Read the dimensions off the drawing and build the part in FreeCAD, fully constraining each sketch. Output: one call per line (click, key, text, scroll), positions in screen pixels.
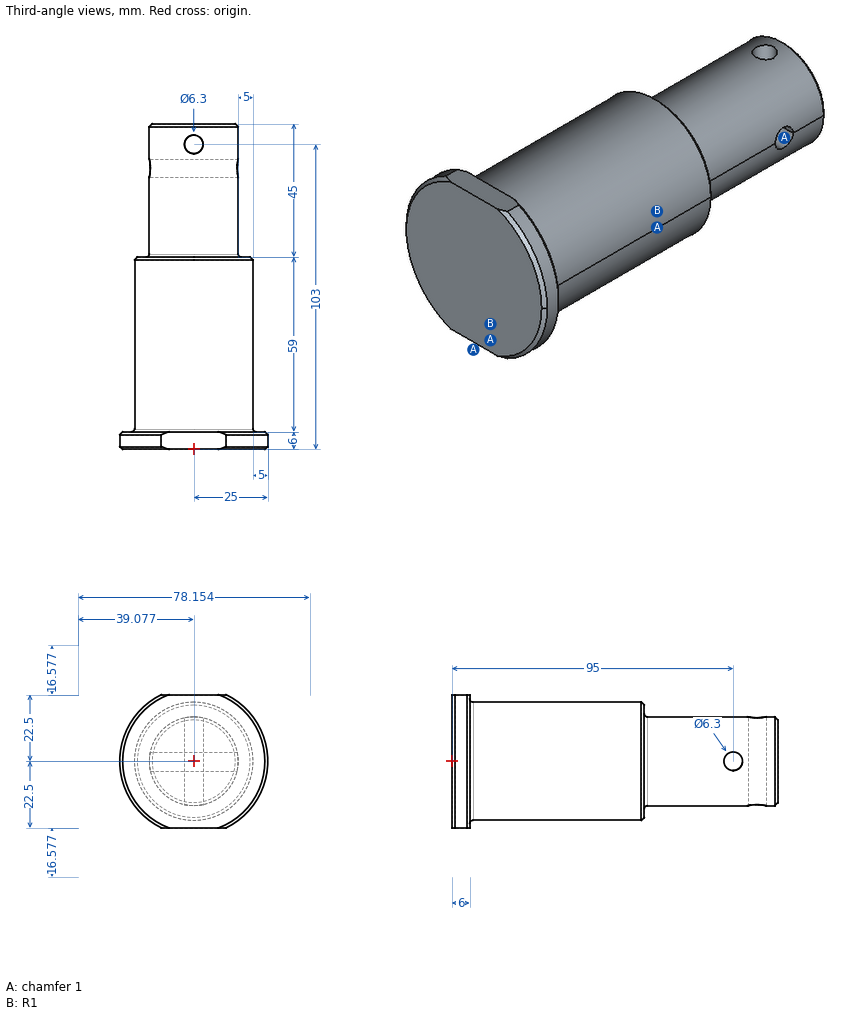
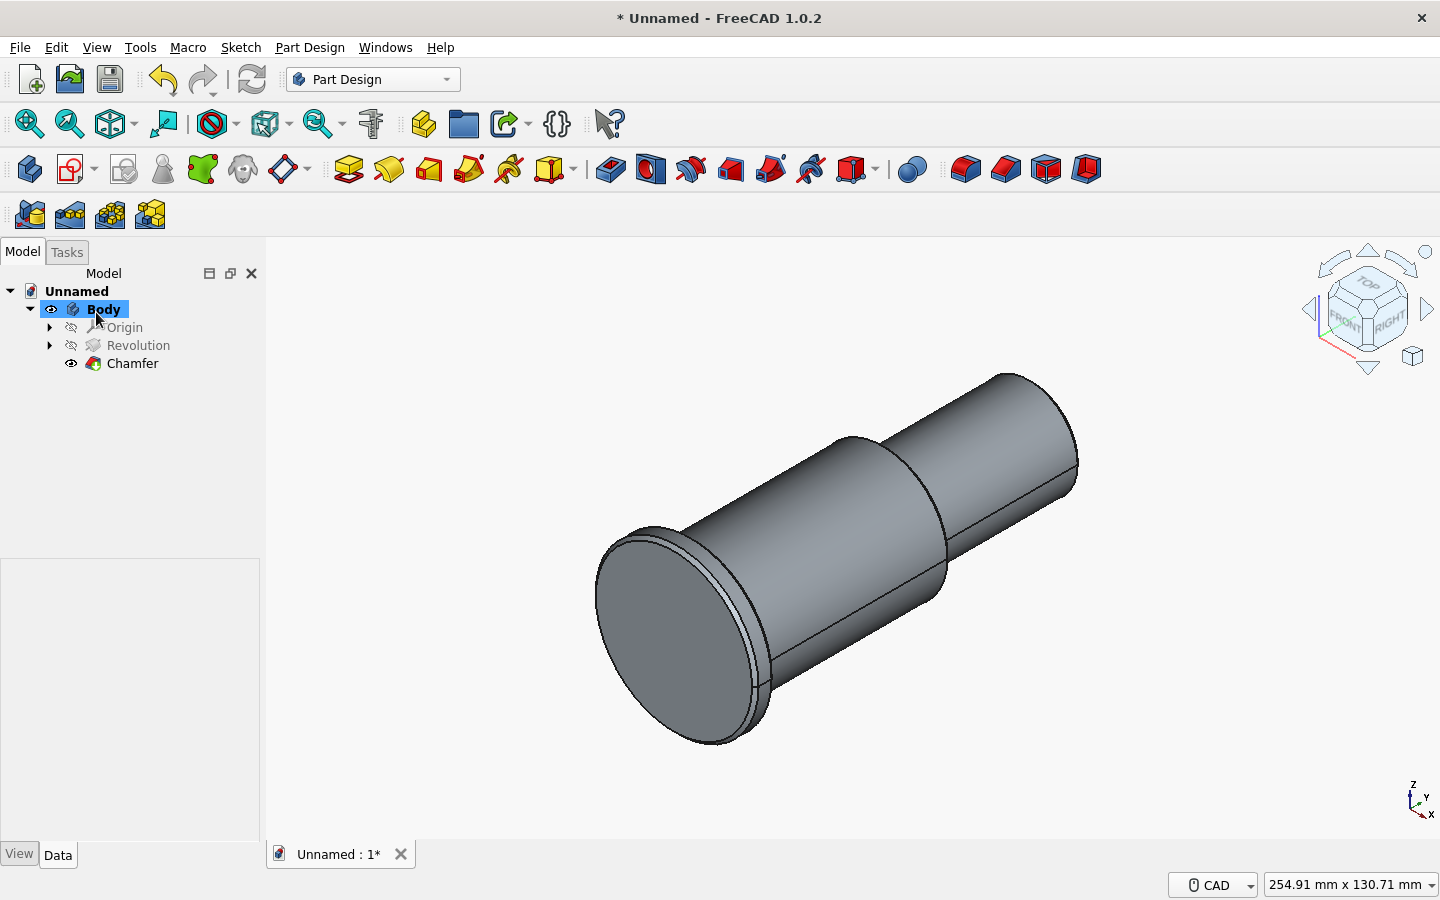
key(2)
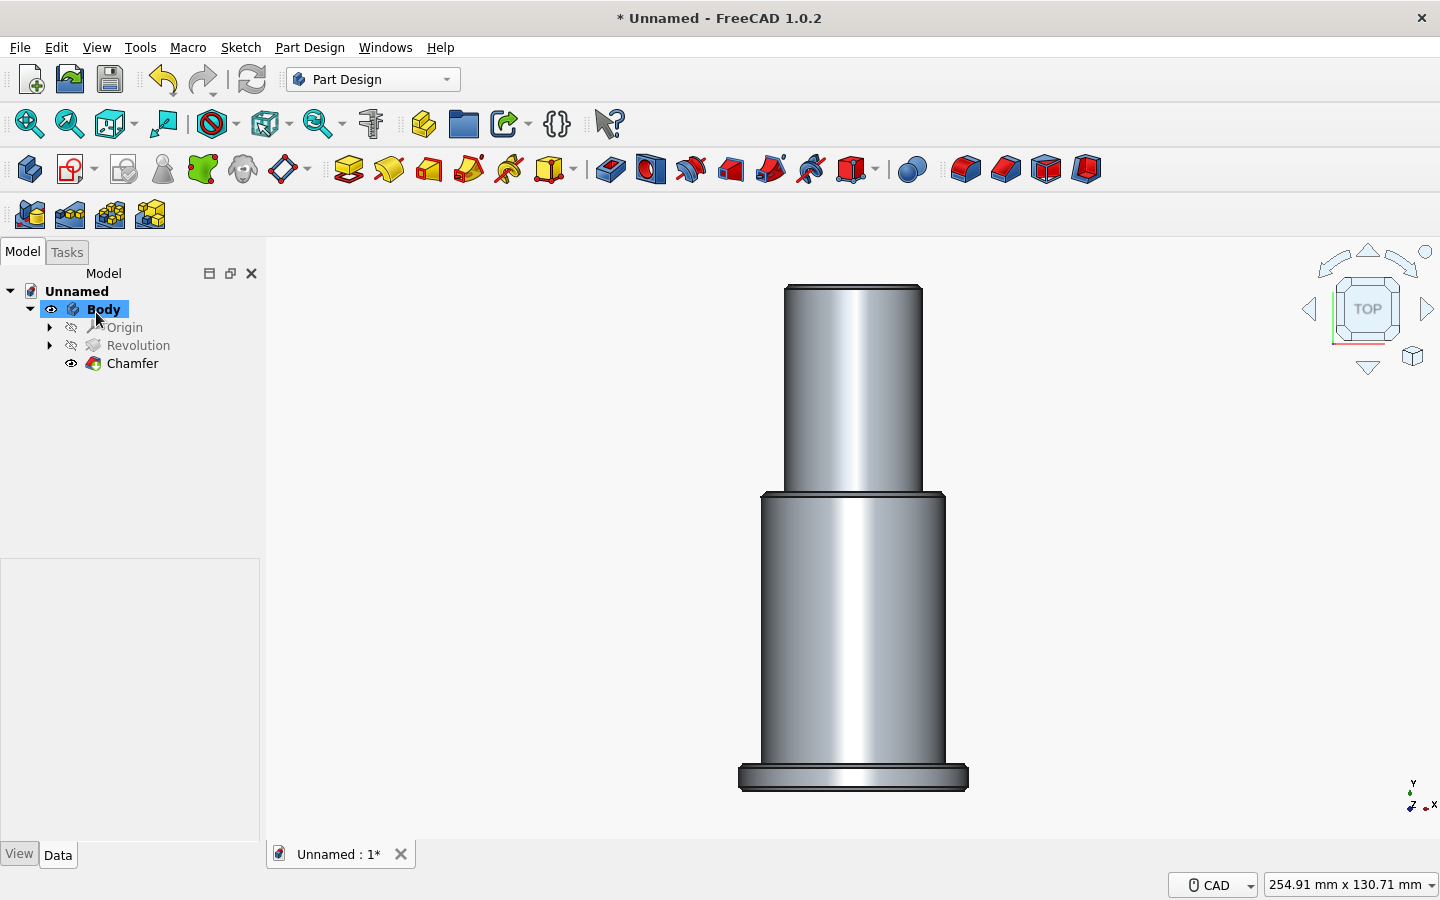
key(1)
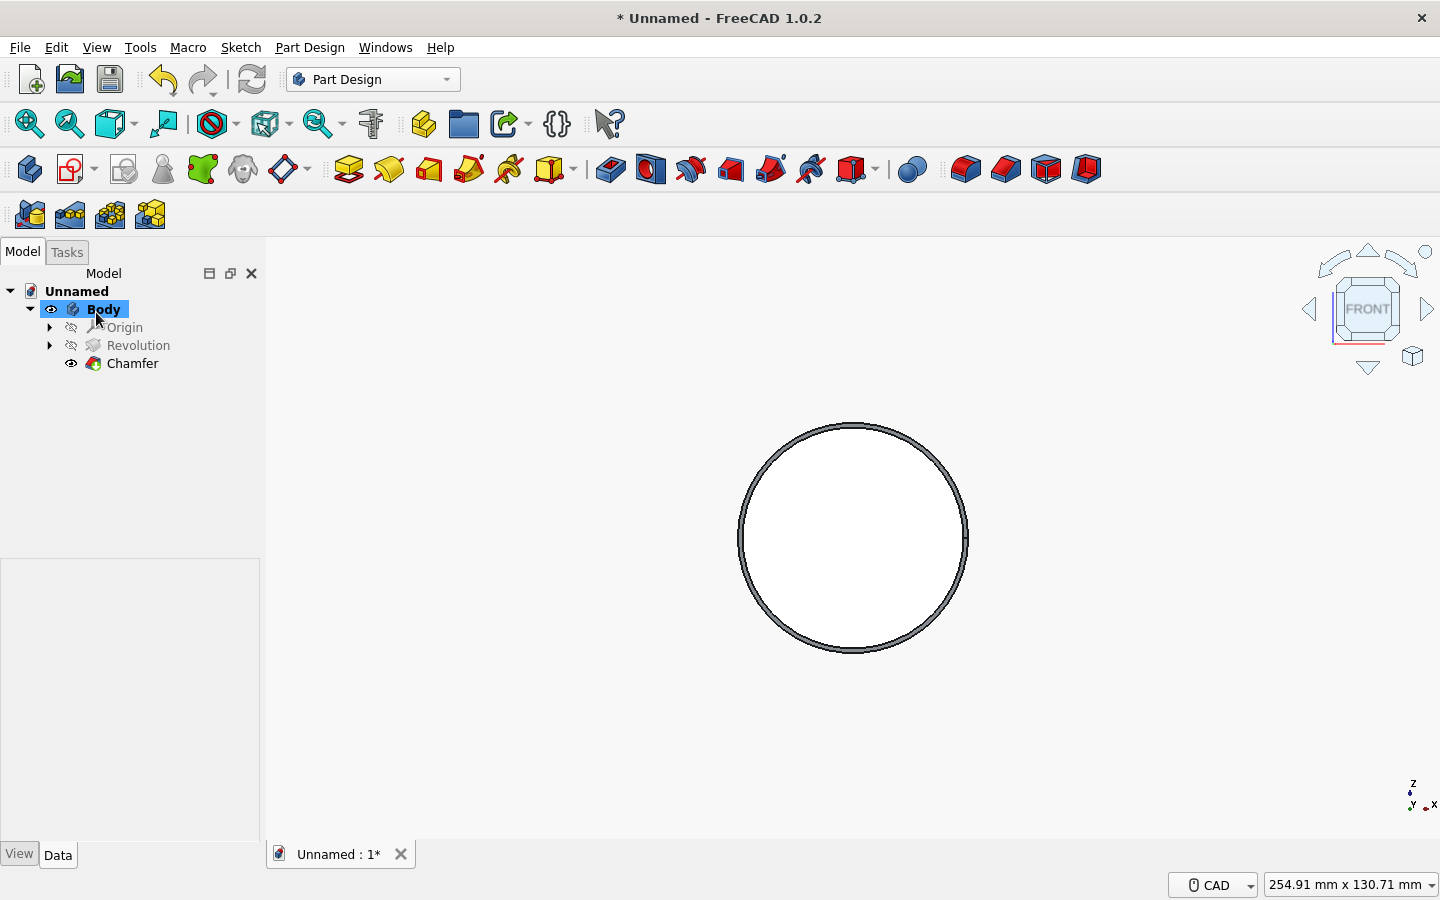
key(v)
key(f)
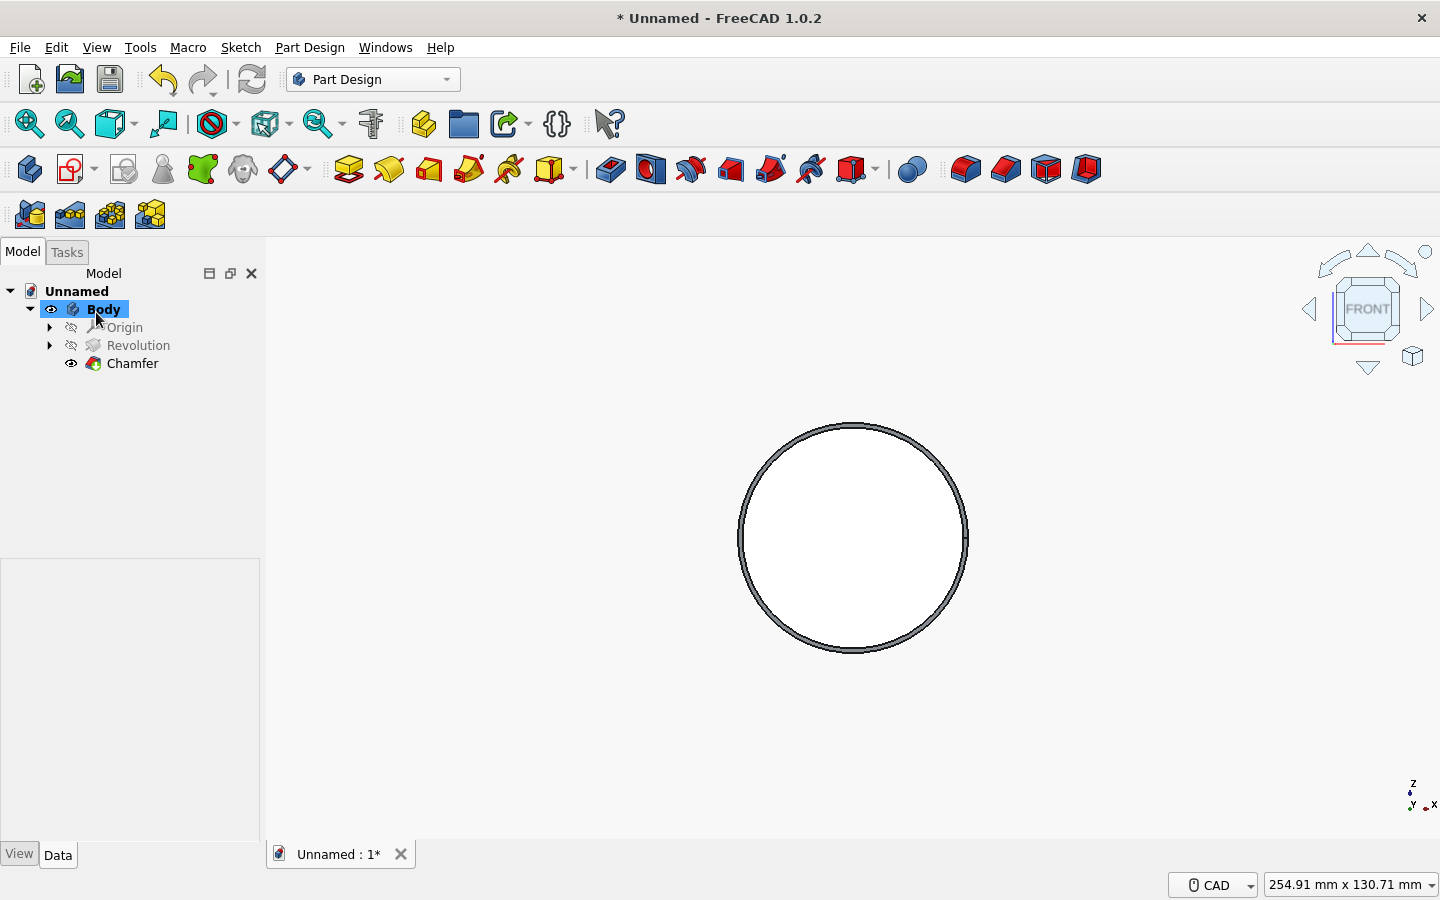
key(3)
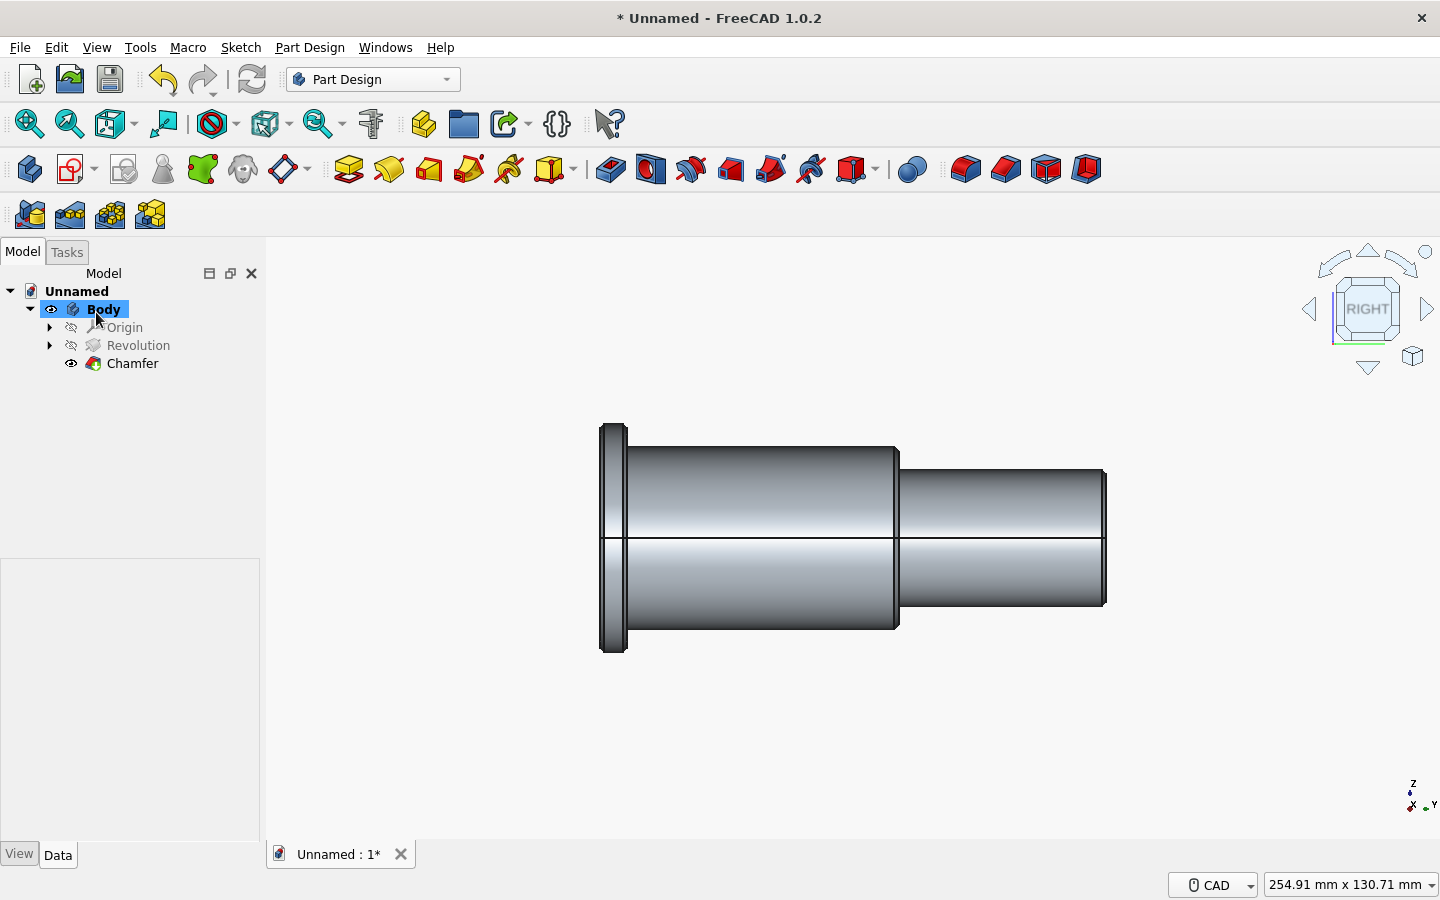
key(v)
key(f)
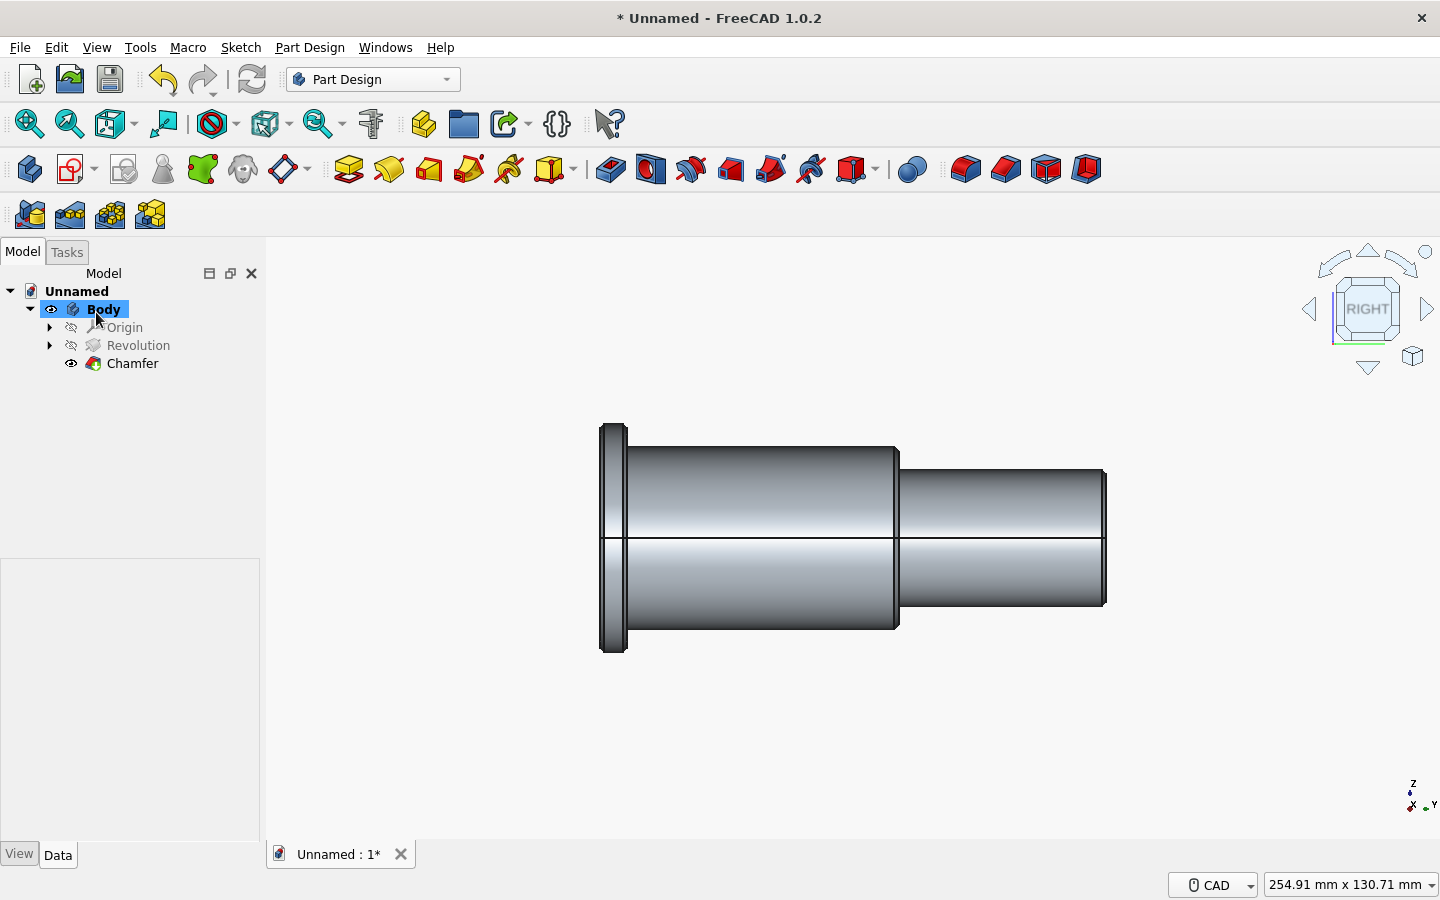
key(5)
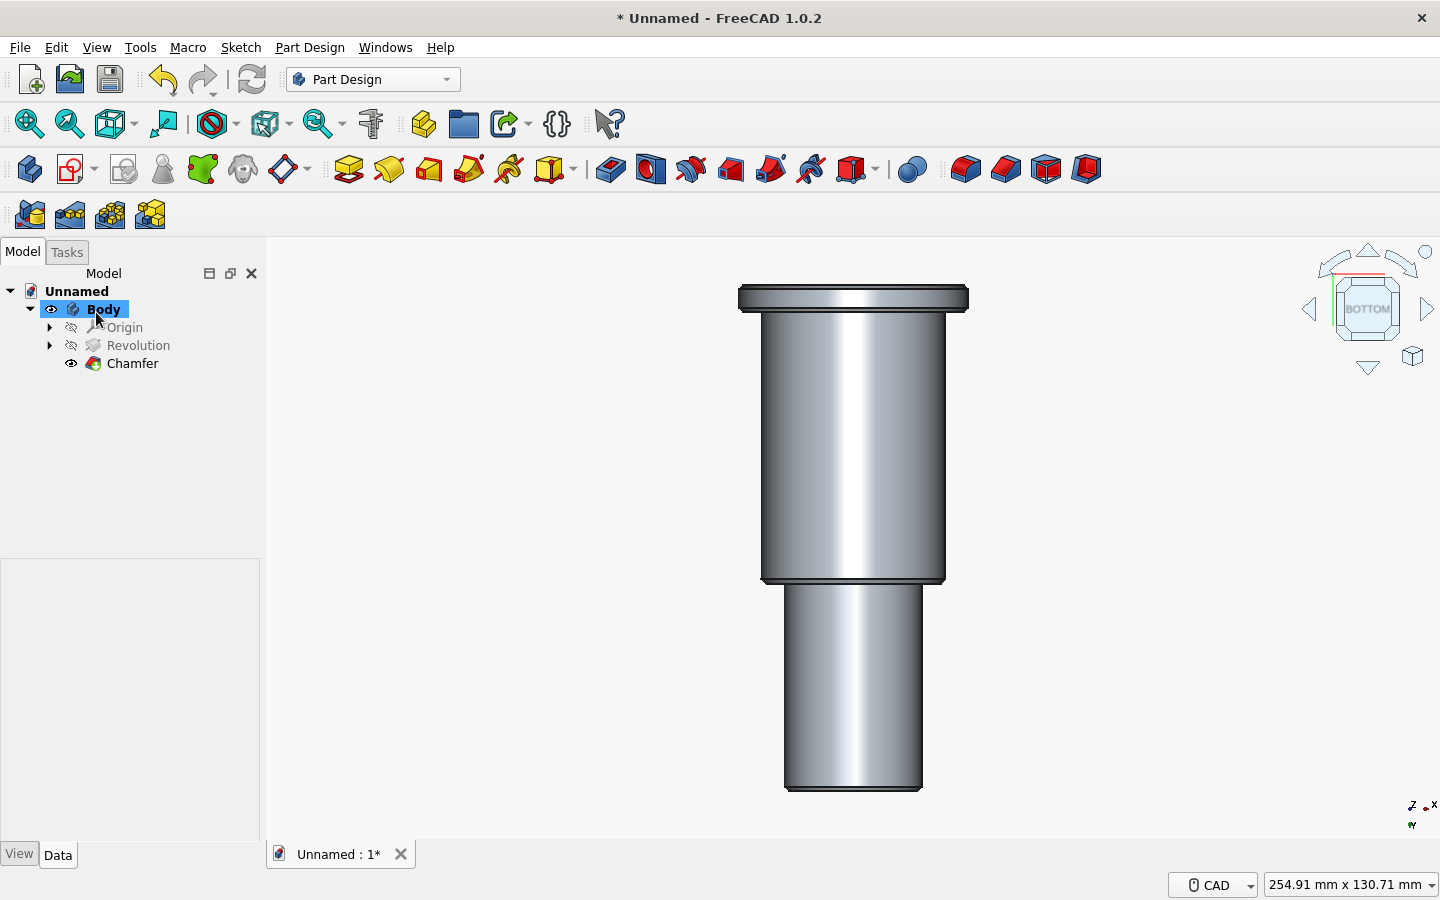
key(4)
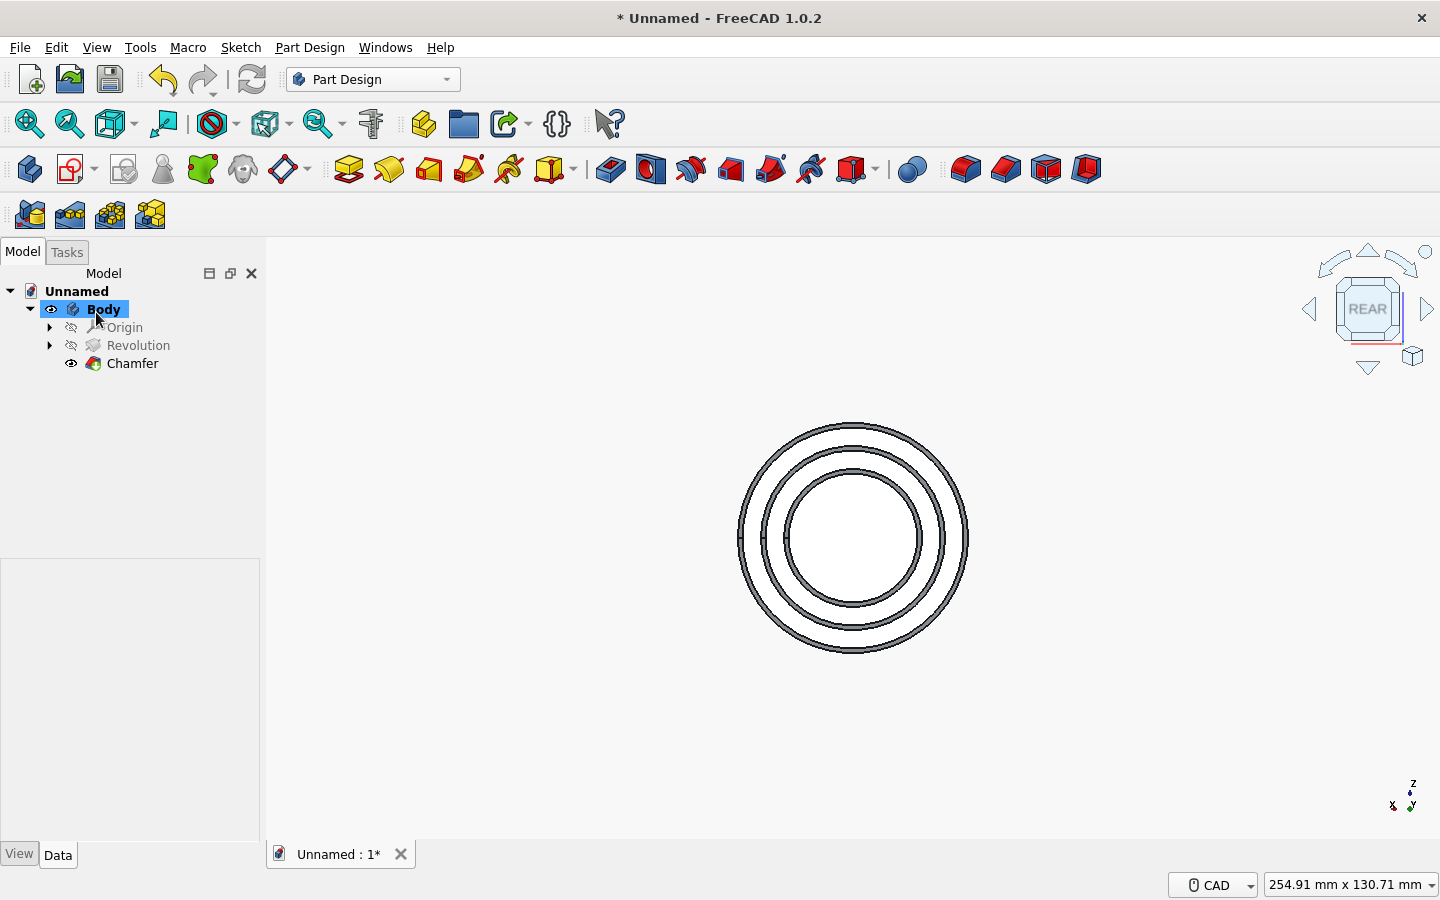
key(v)
key(f)